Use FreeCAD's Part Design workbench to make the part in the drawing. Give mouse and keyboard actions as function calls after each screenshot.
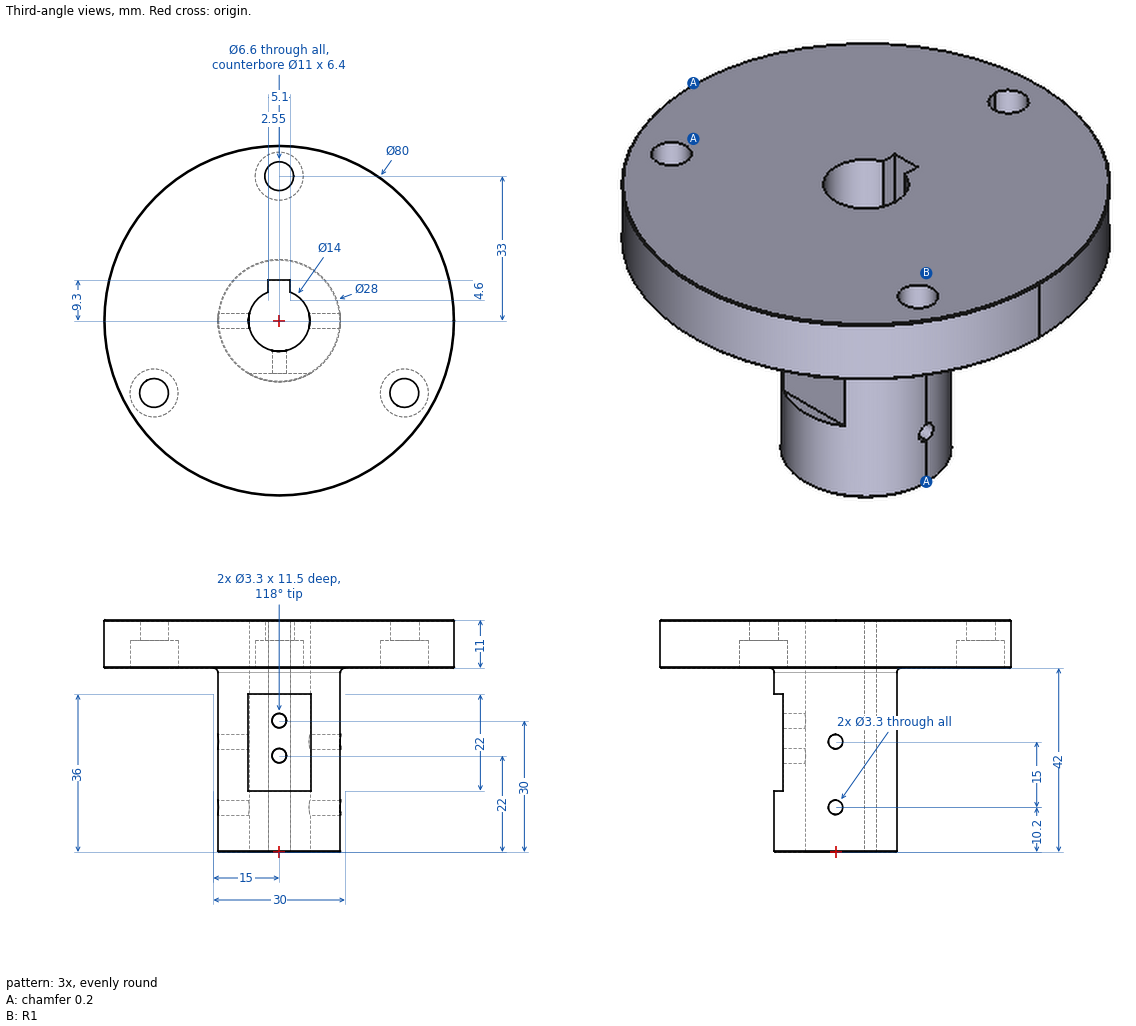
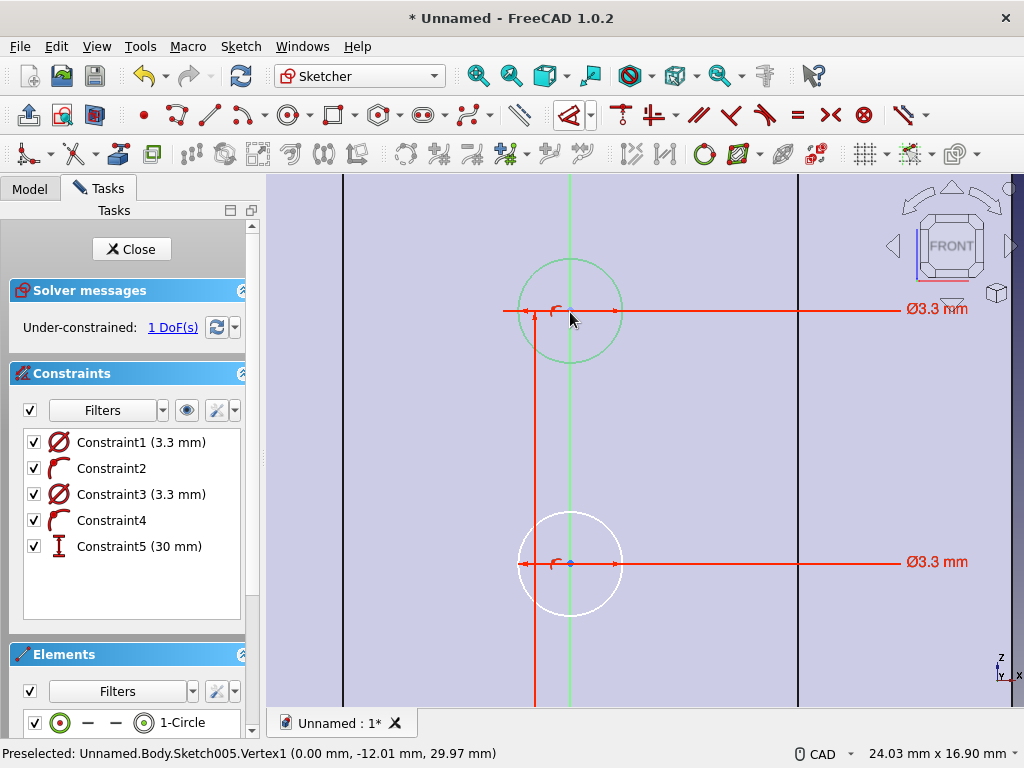
click(570, 564)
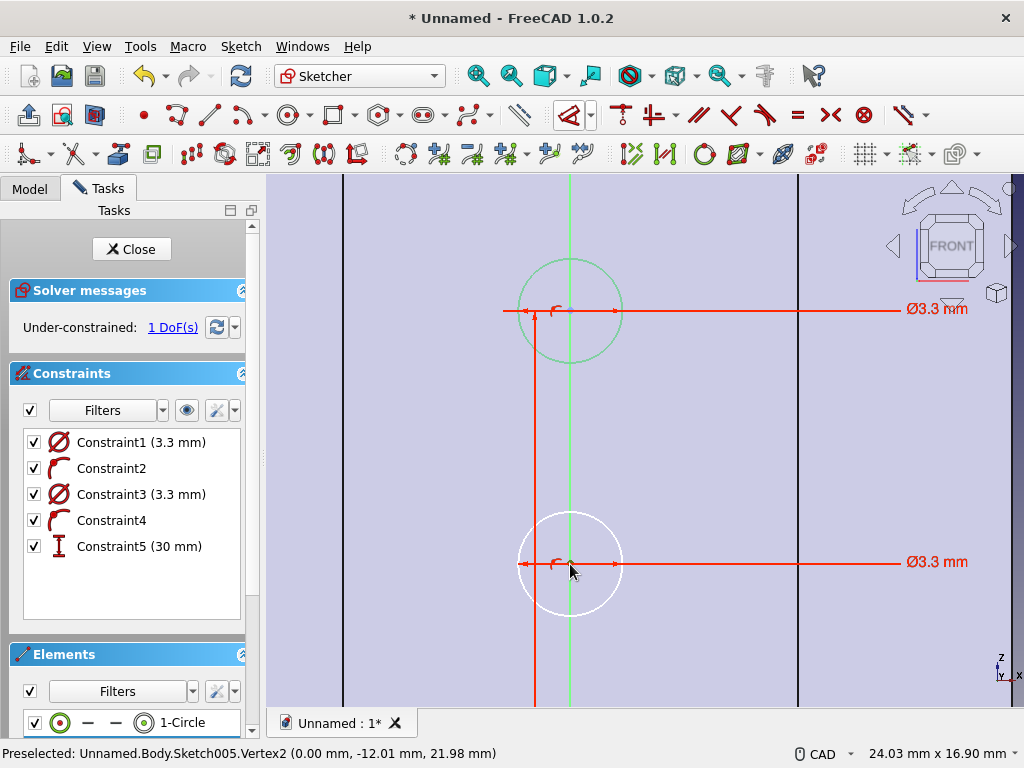
key(i)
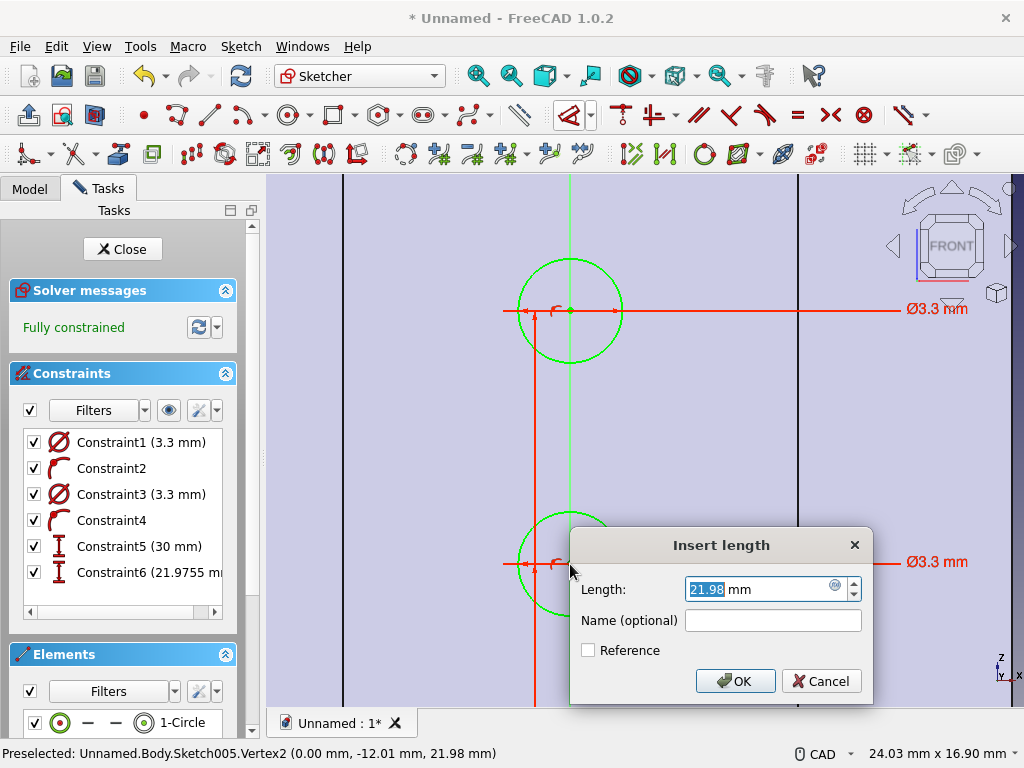
text(22)
key(Return)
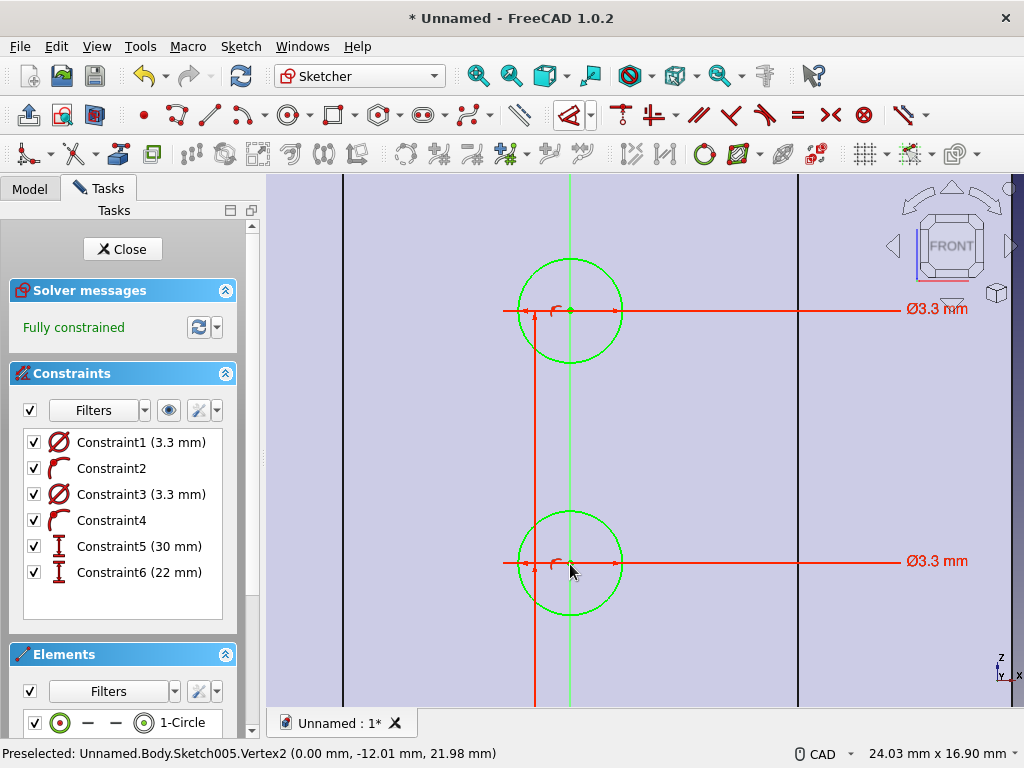
click(123, 249)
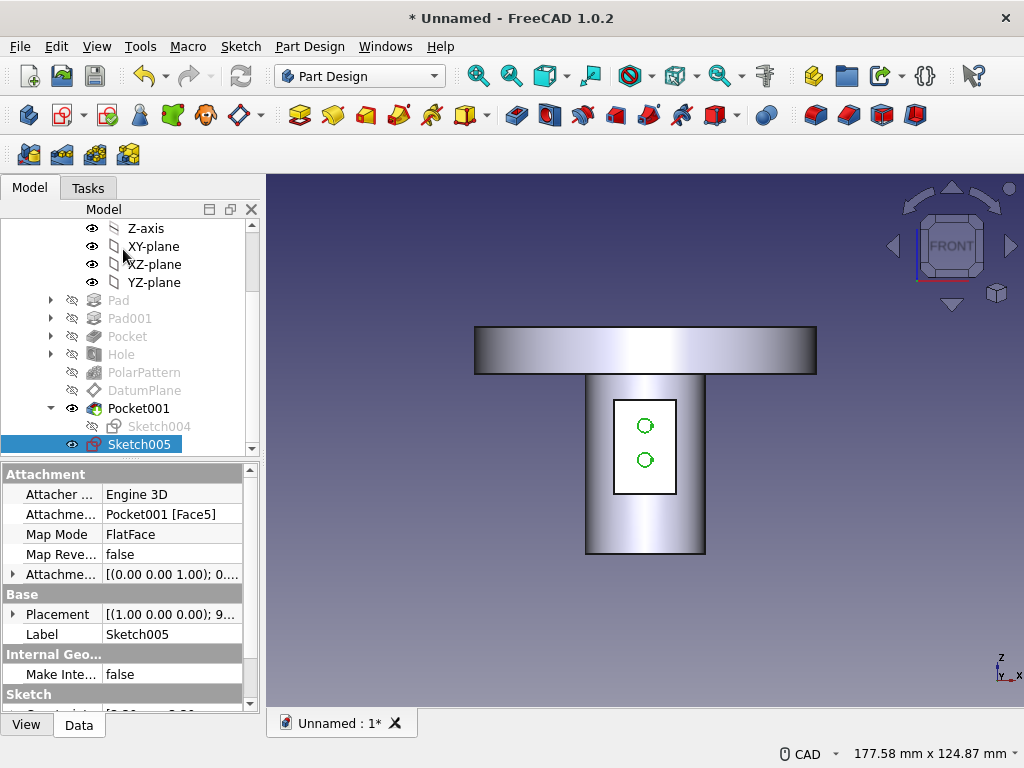
click(550, 116)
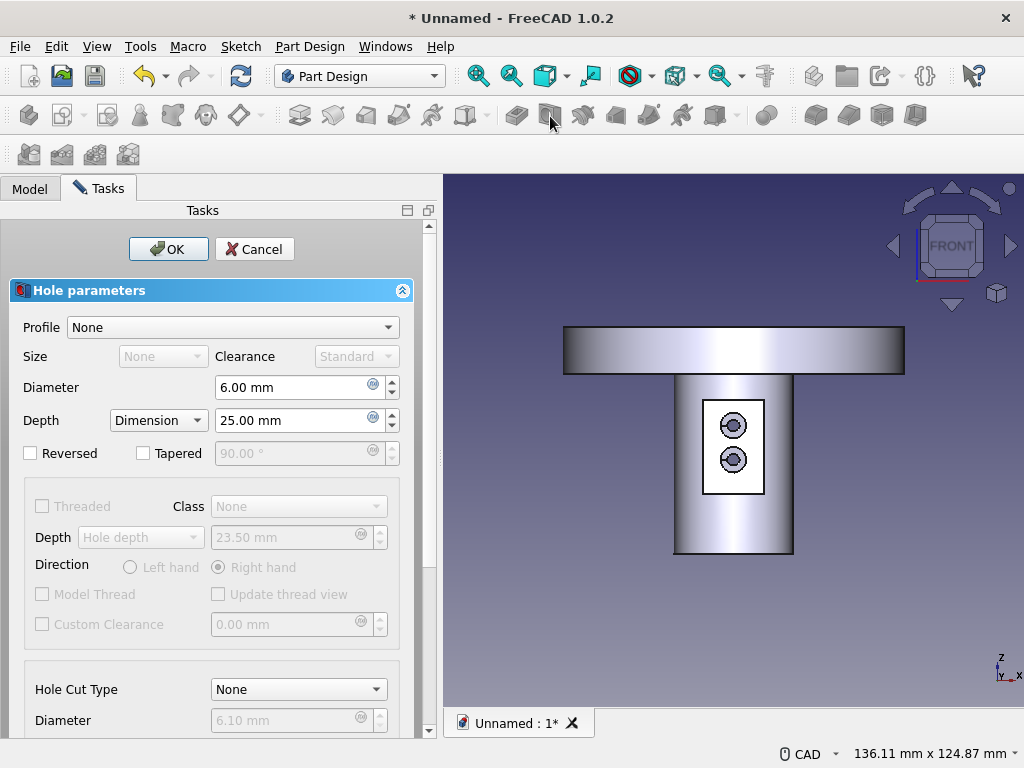
triple_click(300, 388)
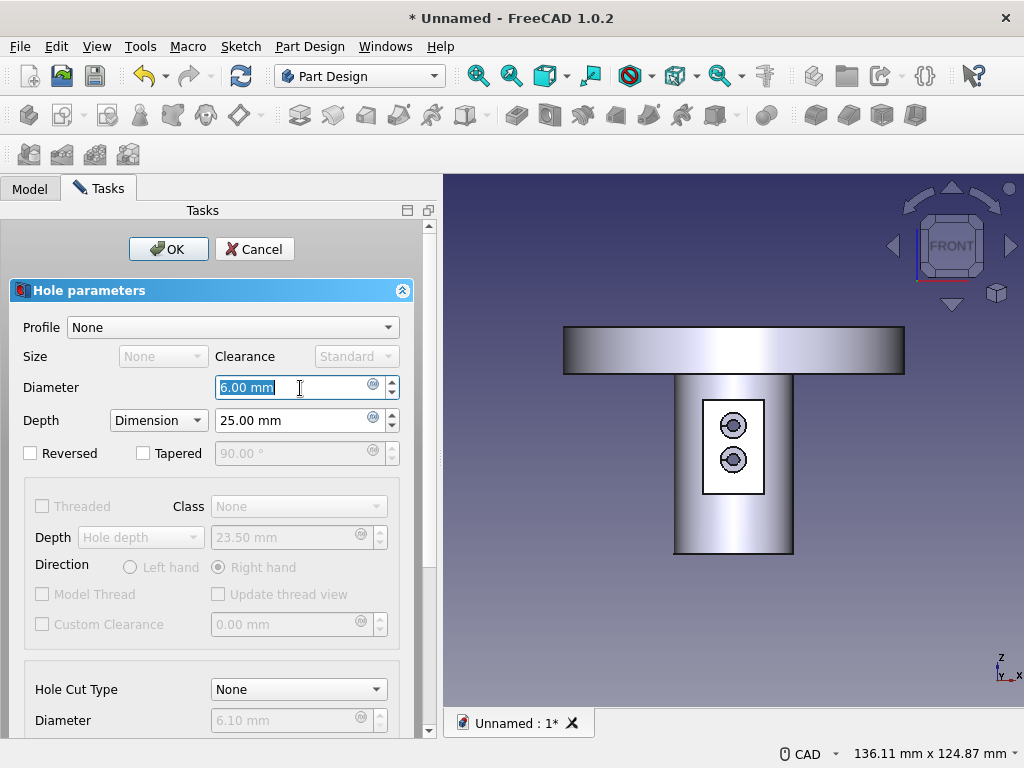
text(3.3)
key(Tab)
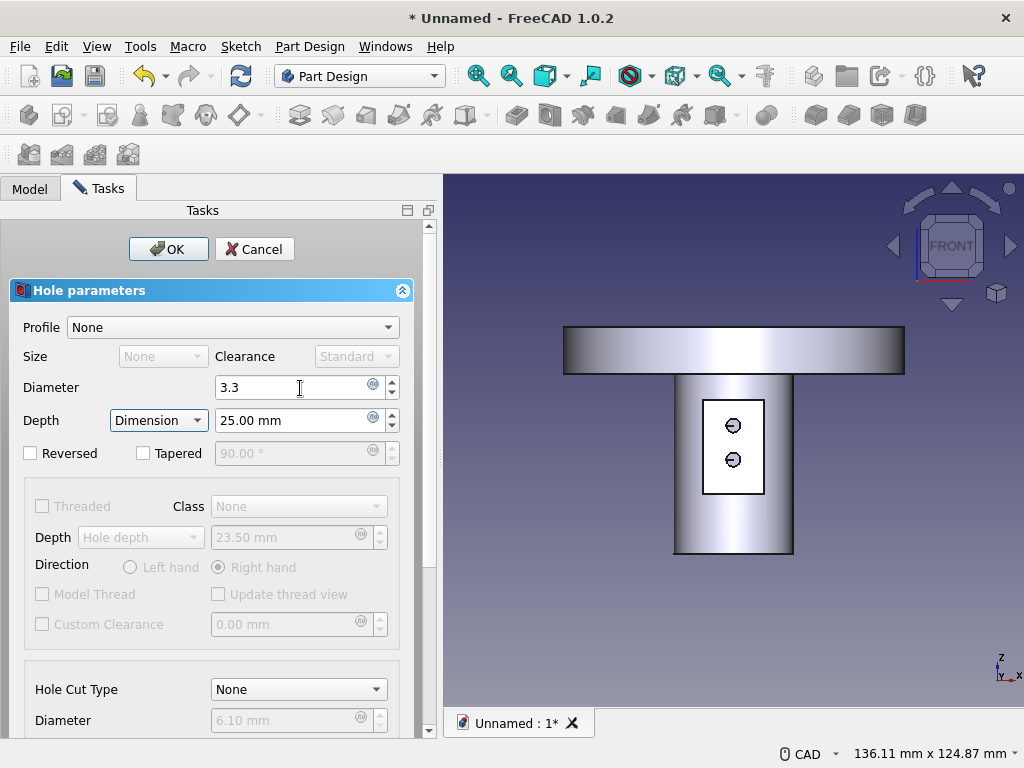
triple_click(300, 420)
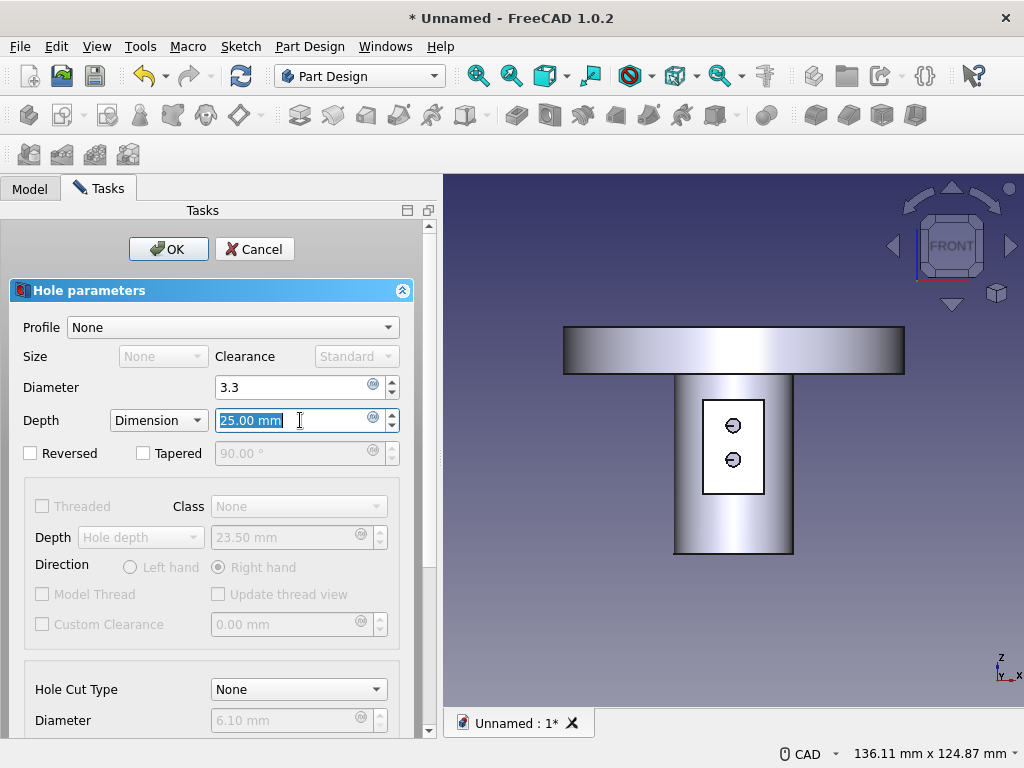
text(11.5)
key(Tab)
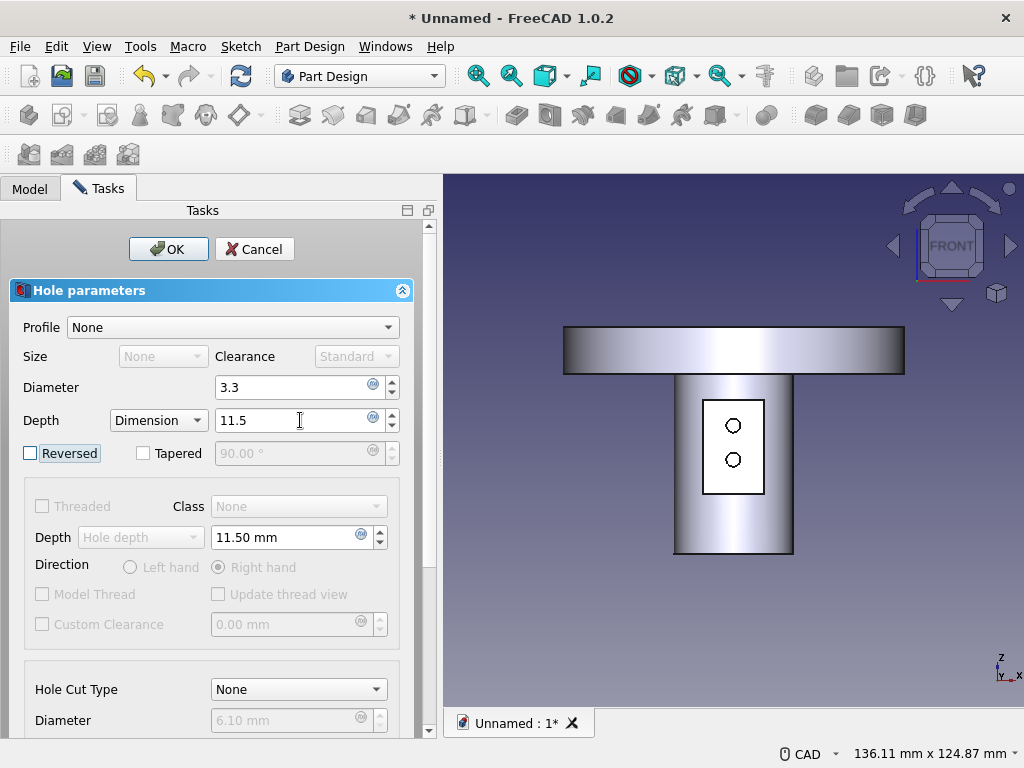
click(169, 249)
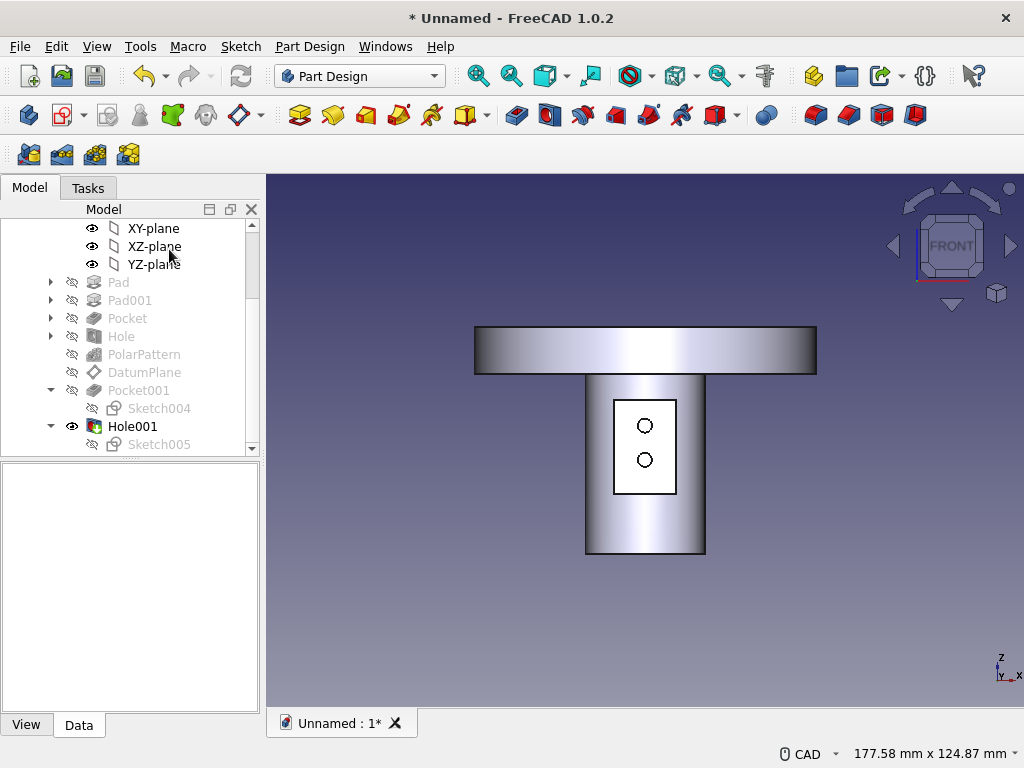
click(62, 116)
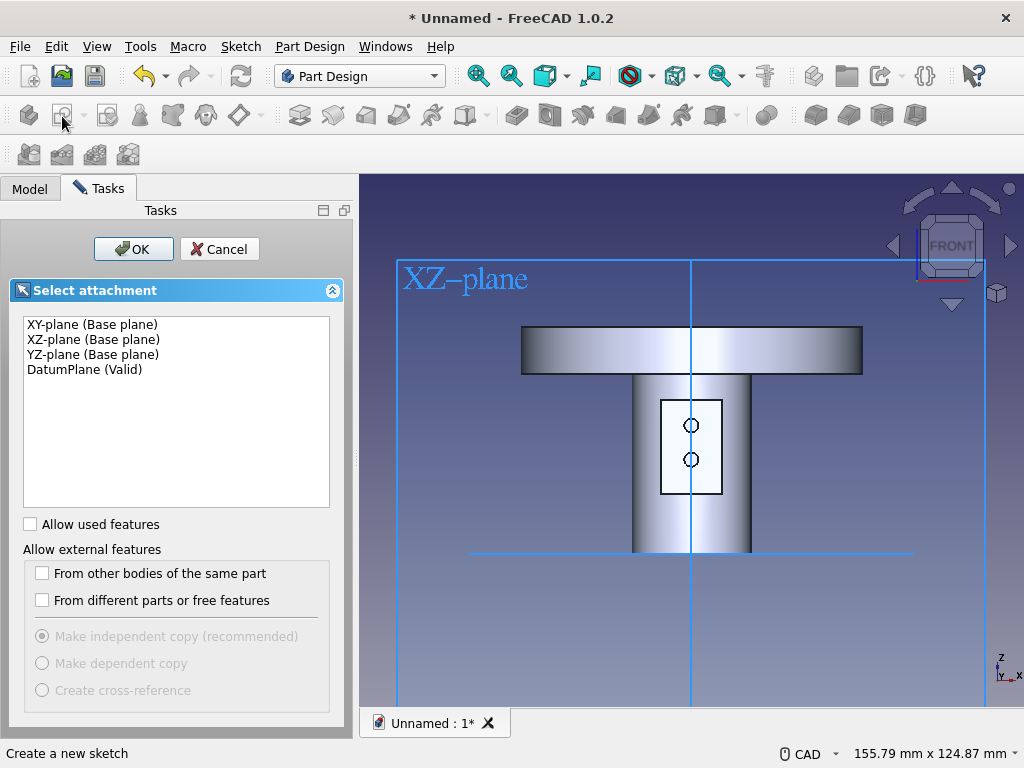
click(84, 324)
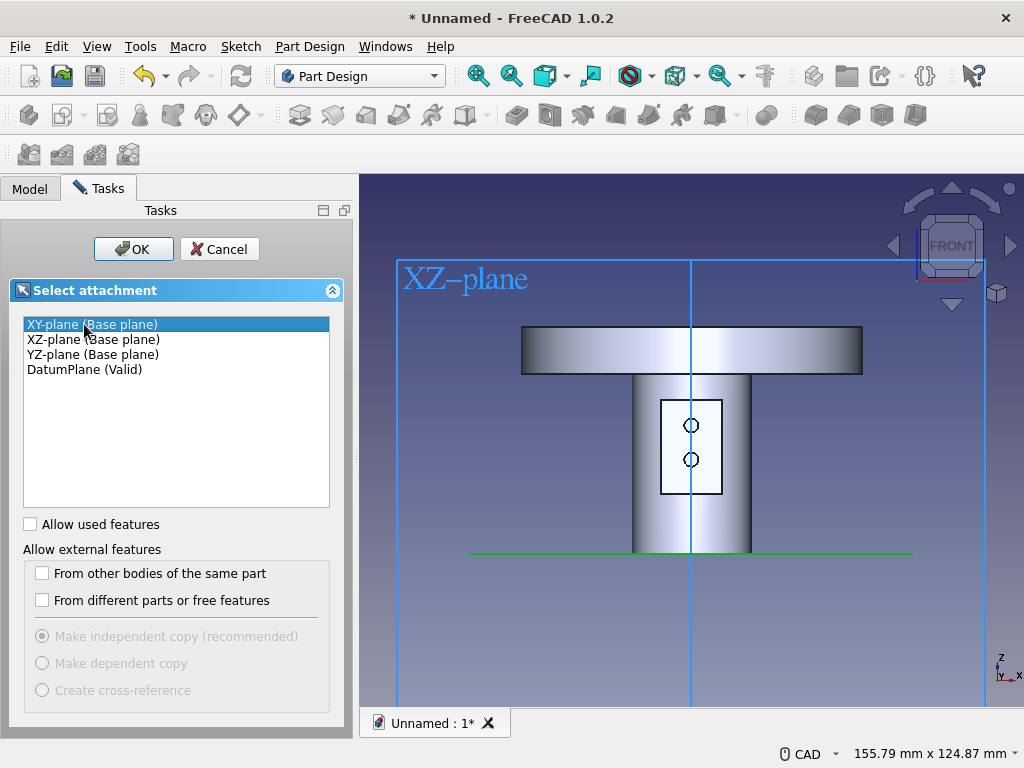
click(134, 249)